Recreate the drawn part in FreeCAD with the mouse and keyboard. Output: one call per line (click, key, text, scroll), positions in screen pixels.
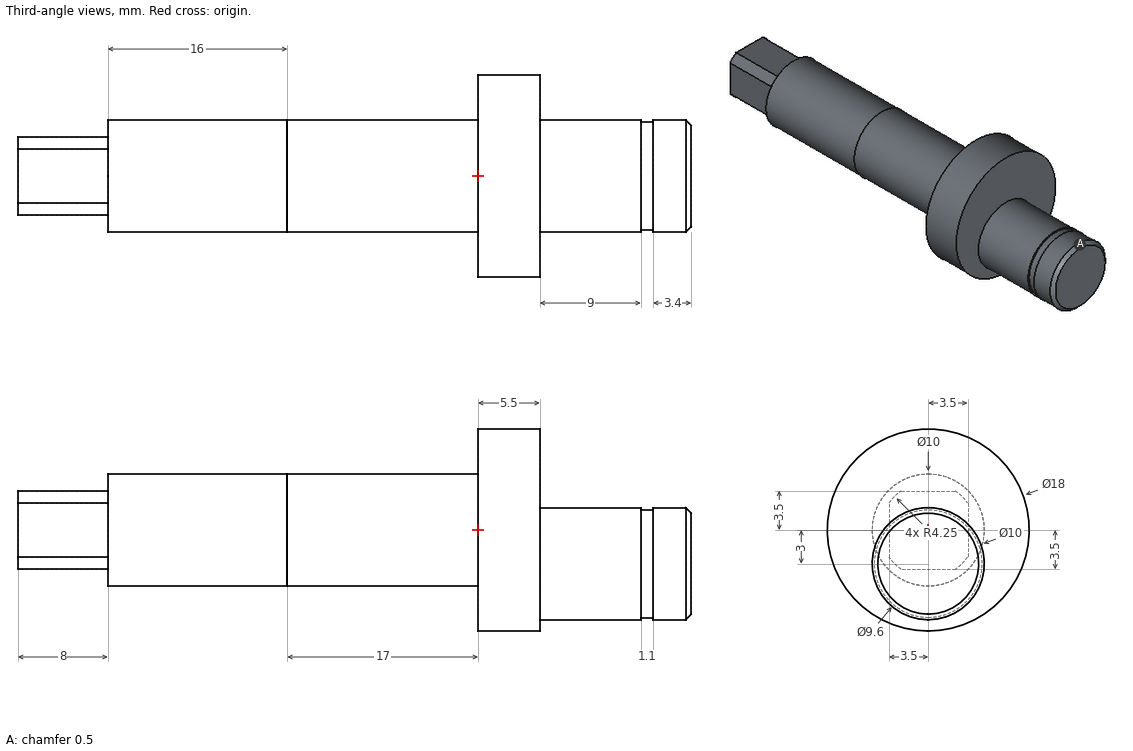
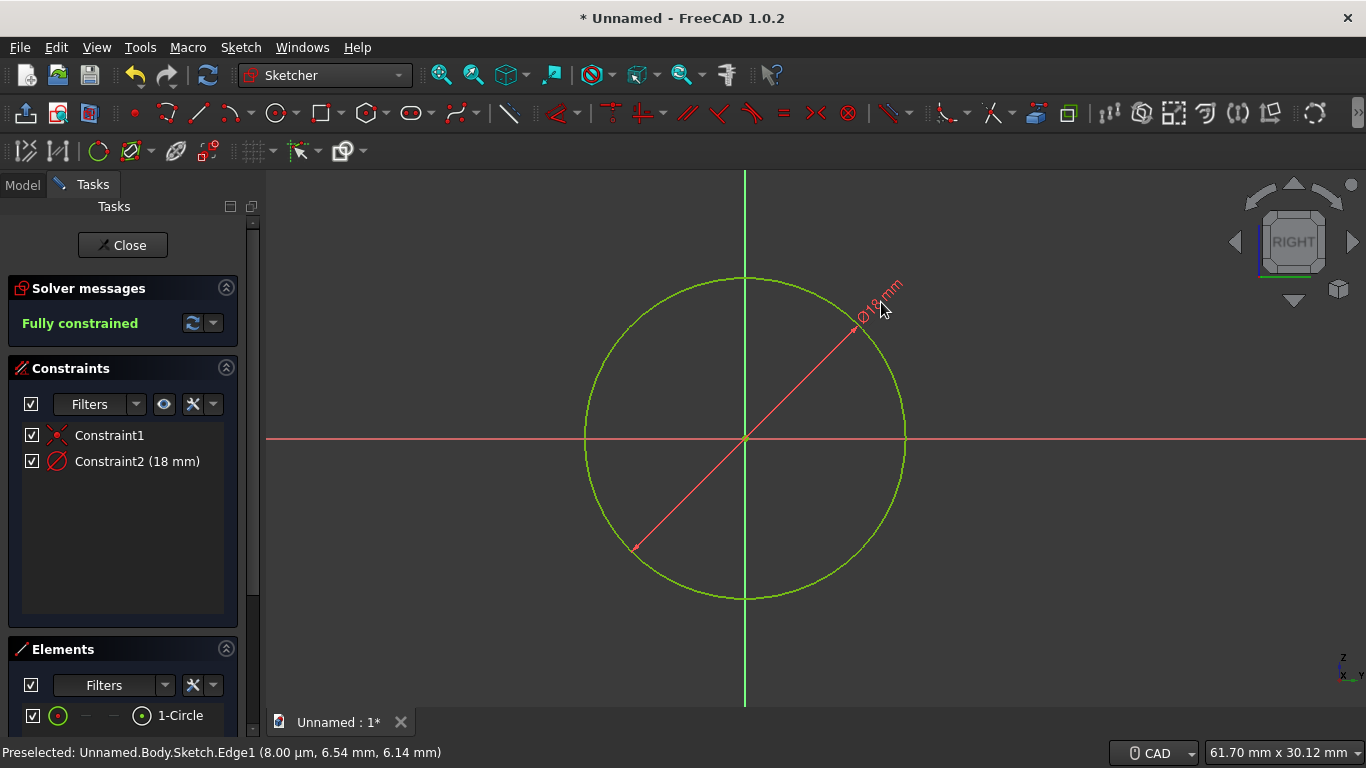
click(123, 245)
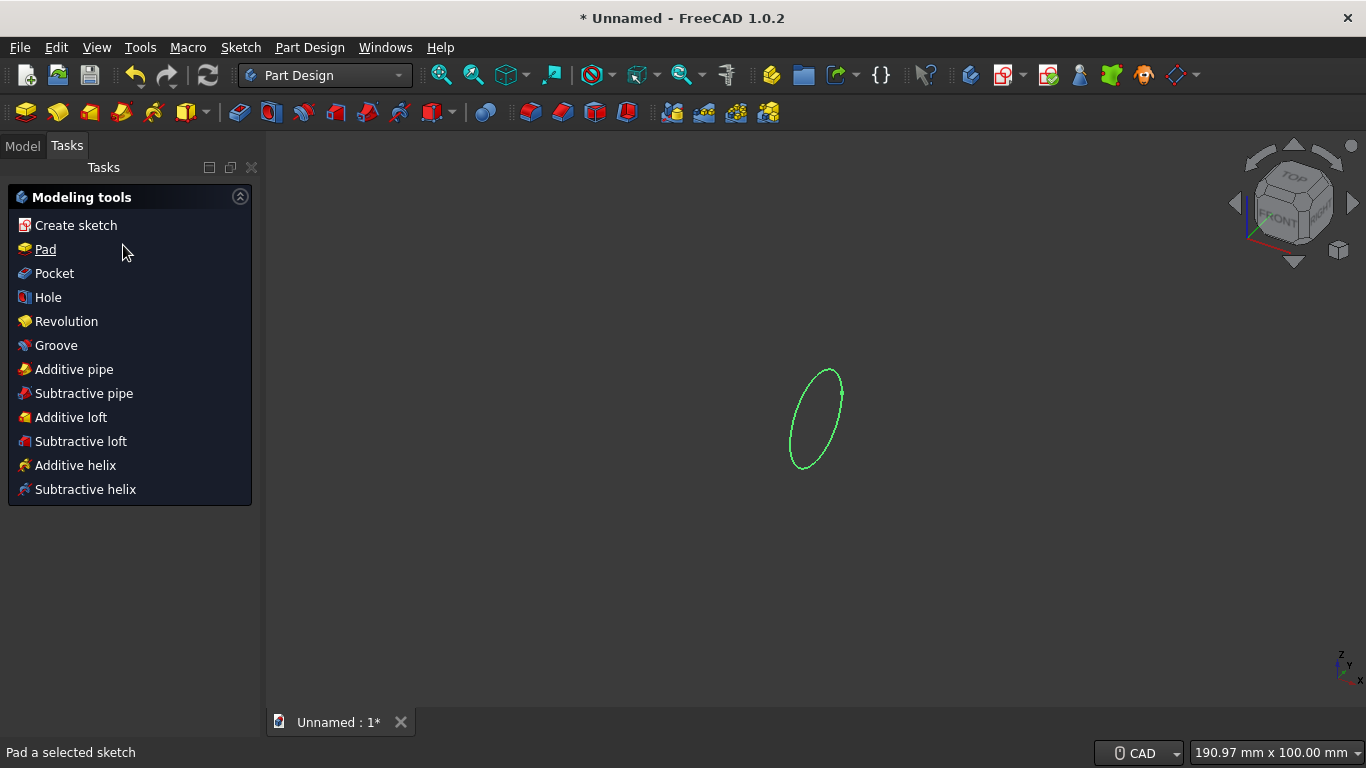
click(26, 112)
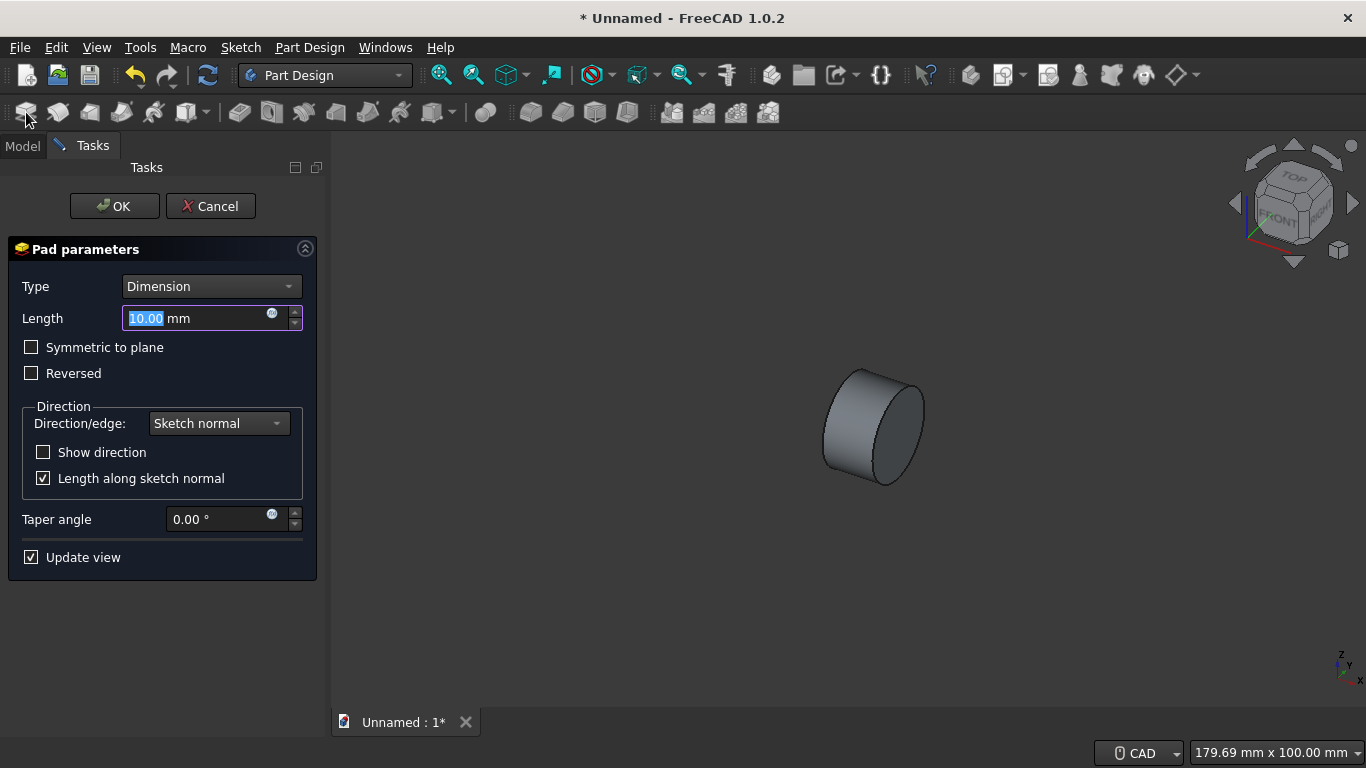
text(5.5)
key(Tab)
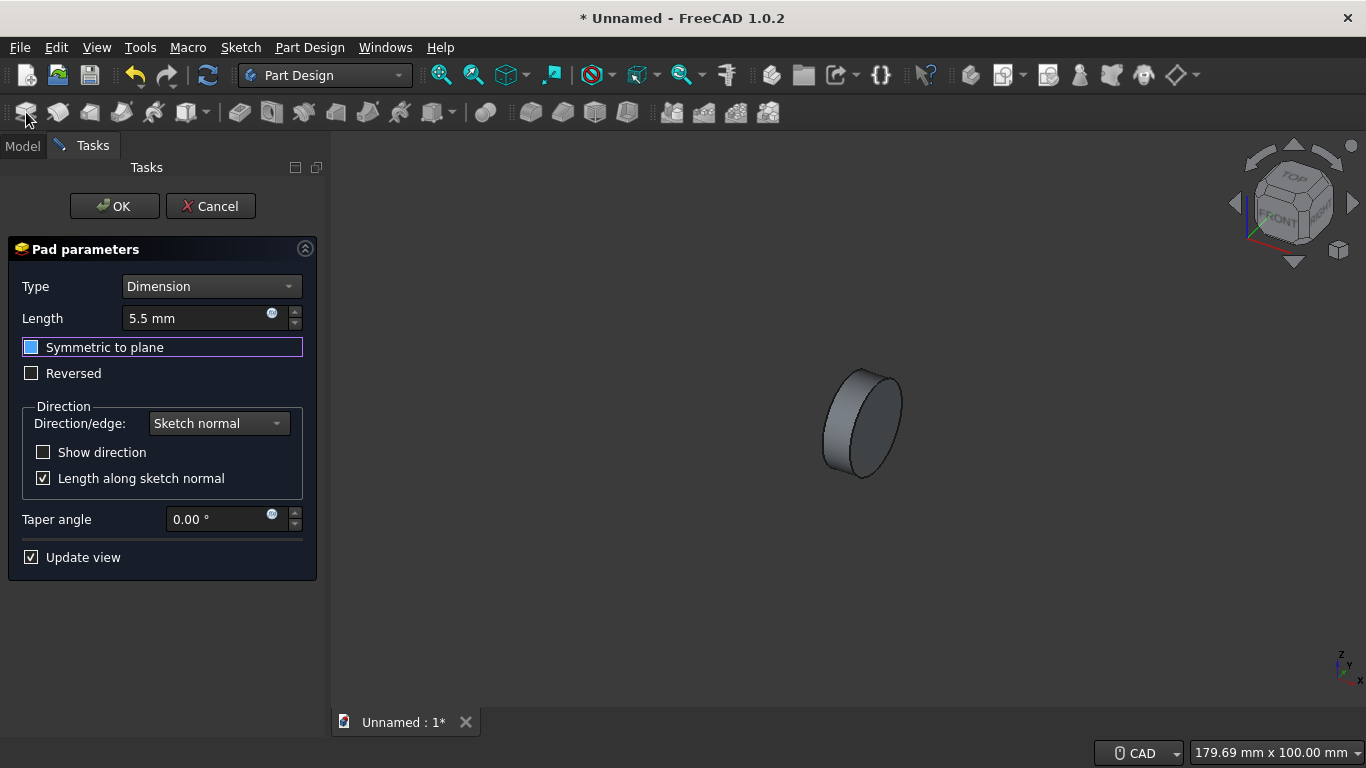
click(115, 206)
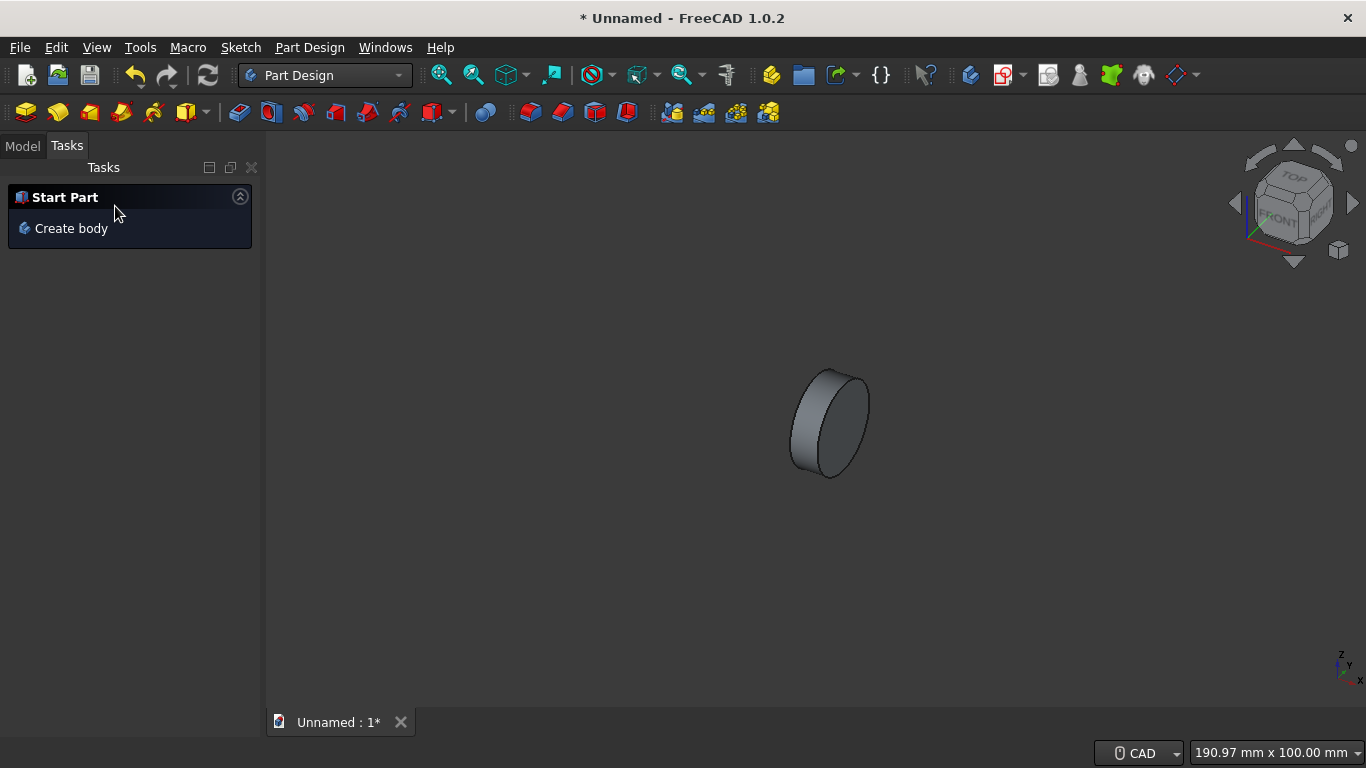
key(v)
key(f)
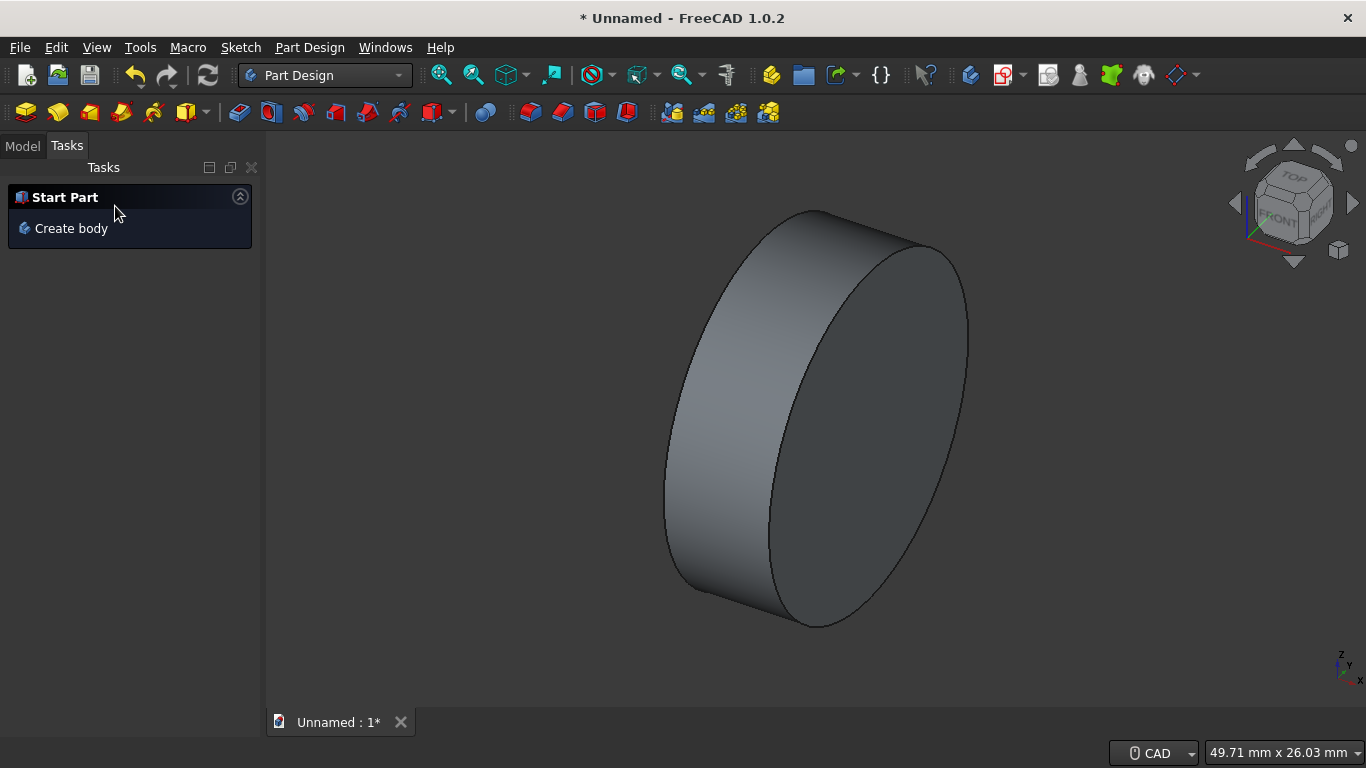
click(869, 436)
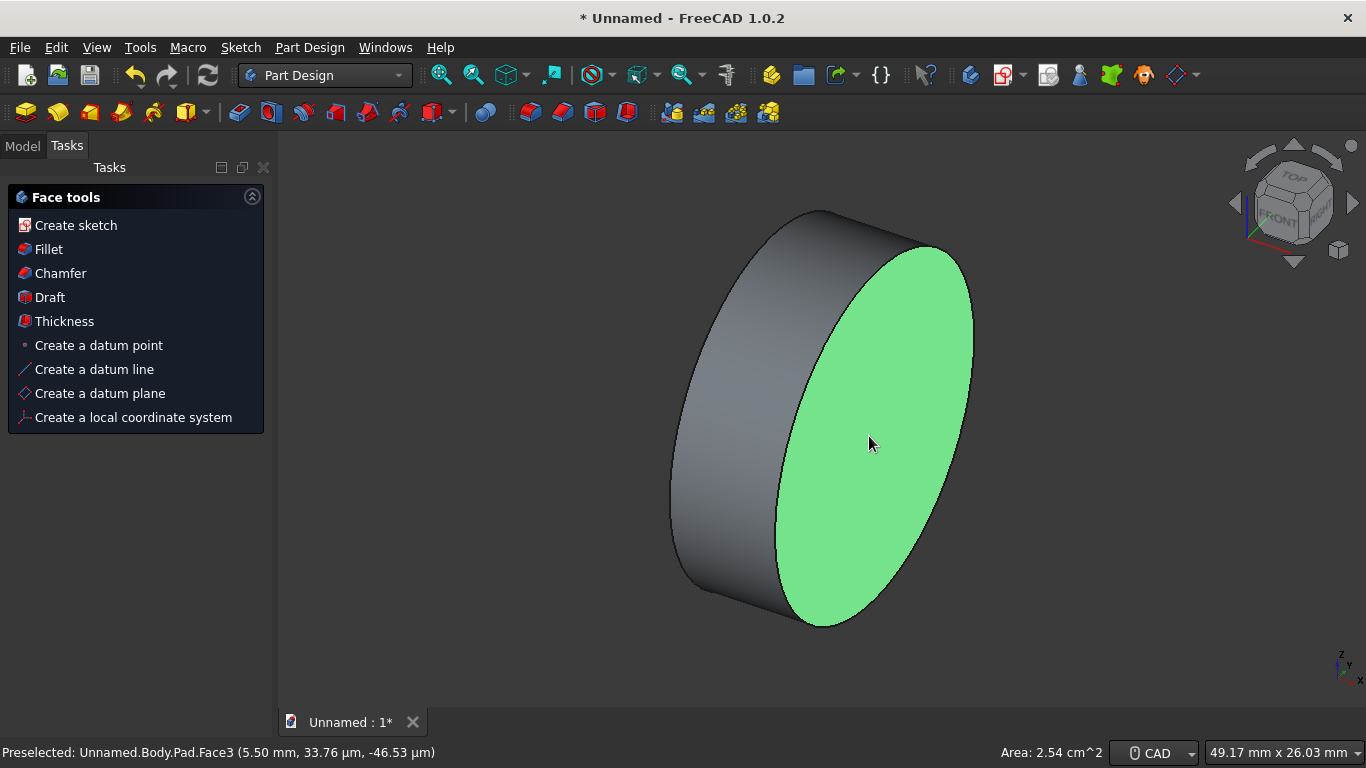
click(1004, 76)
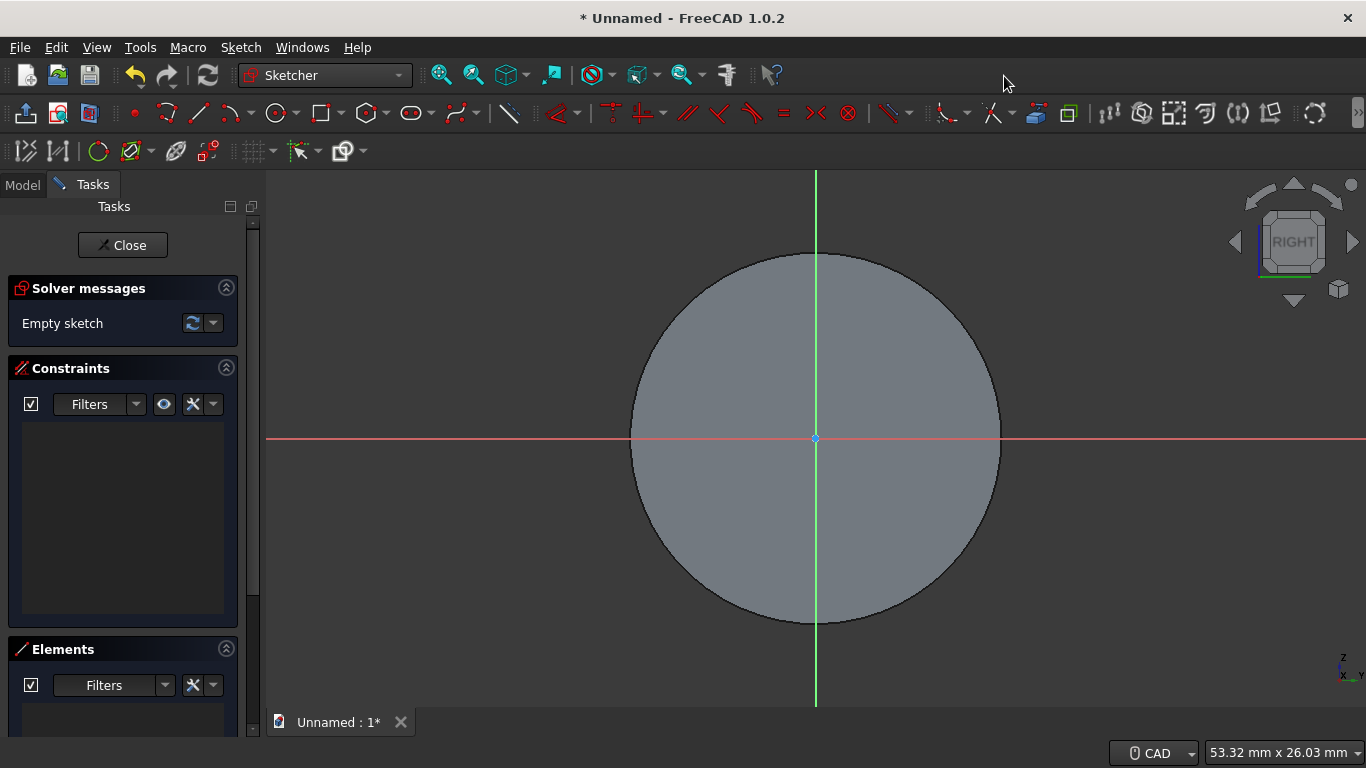
scroll(955, 626, up, 2)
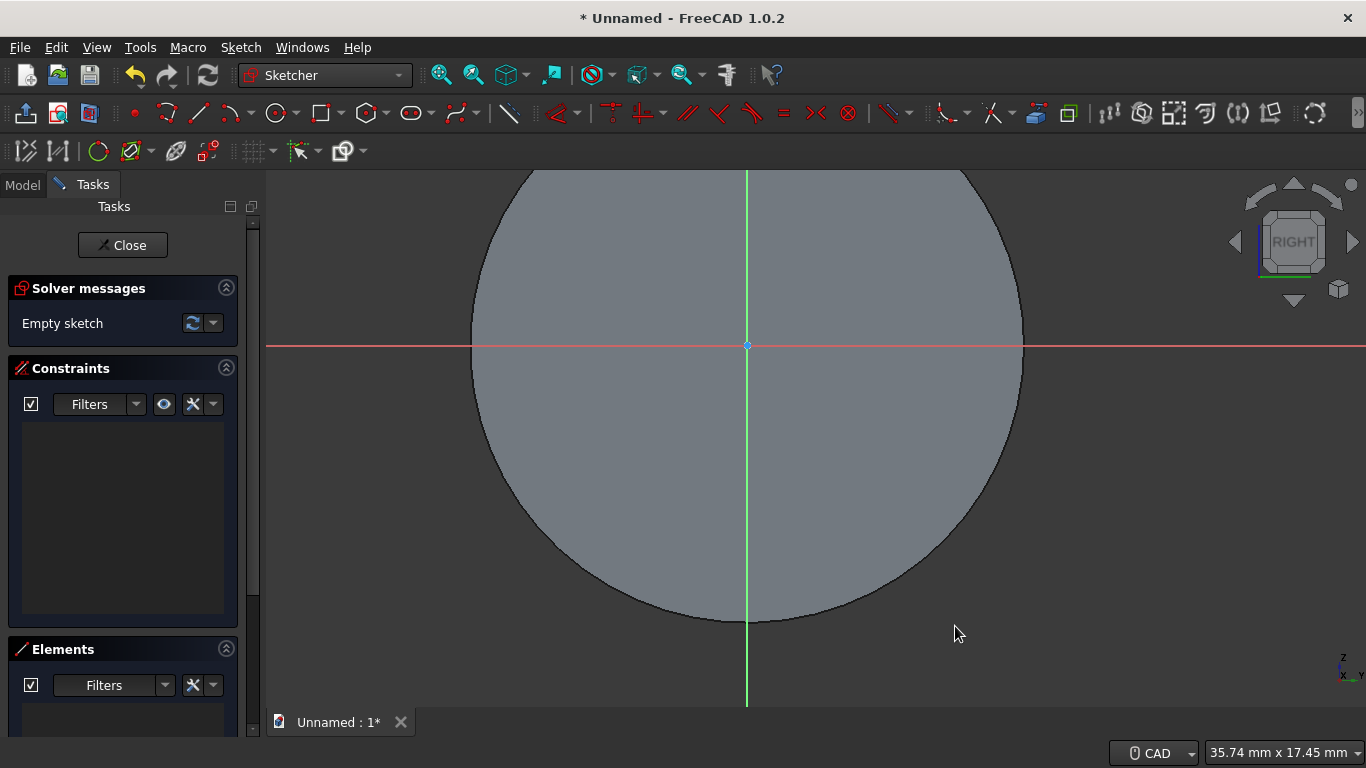
key(g)
key(c)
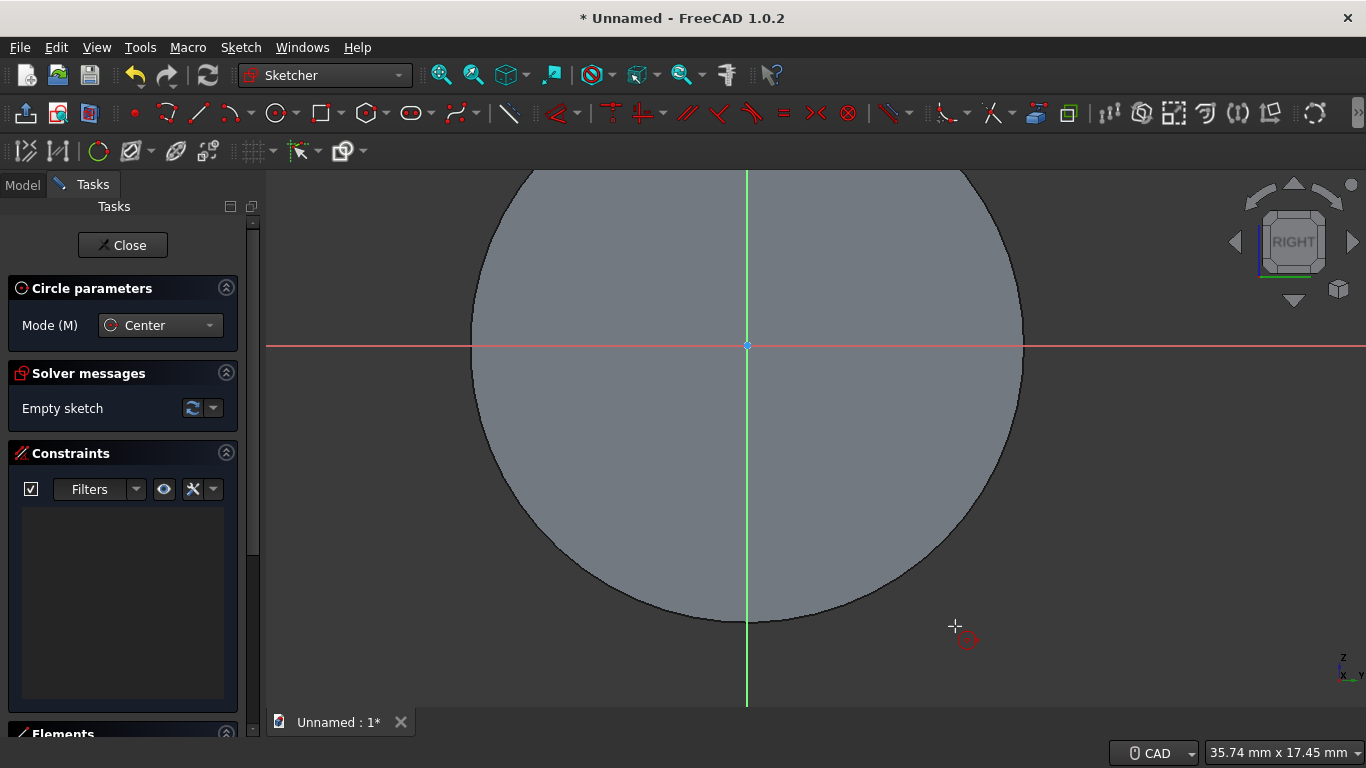
click(747, 438)
click(856, 329)
key(Escape)